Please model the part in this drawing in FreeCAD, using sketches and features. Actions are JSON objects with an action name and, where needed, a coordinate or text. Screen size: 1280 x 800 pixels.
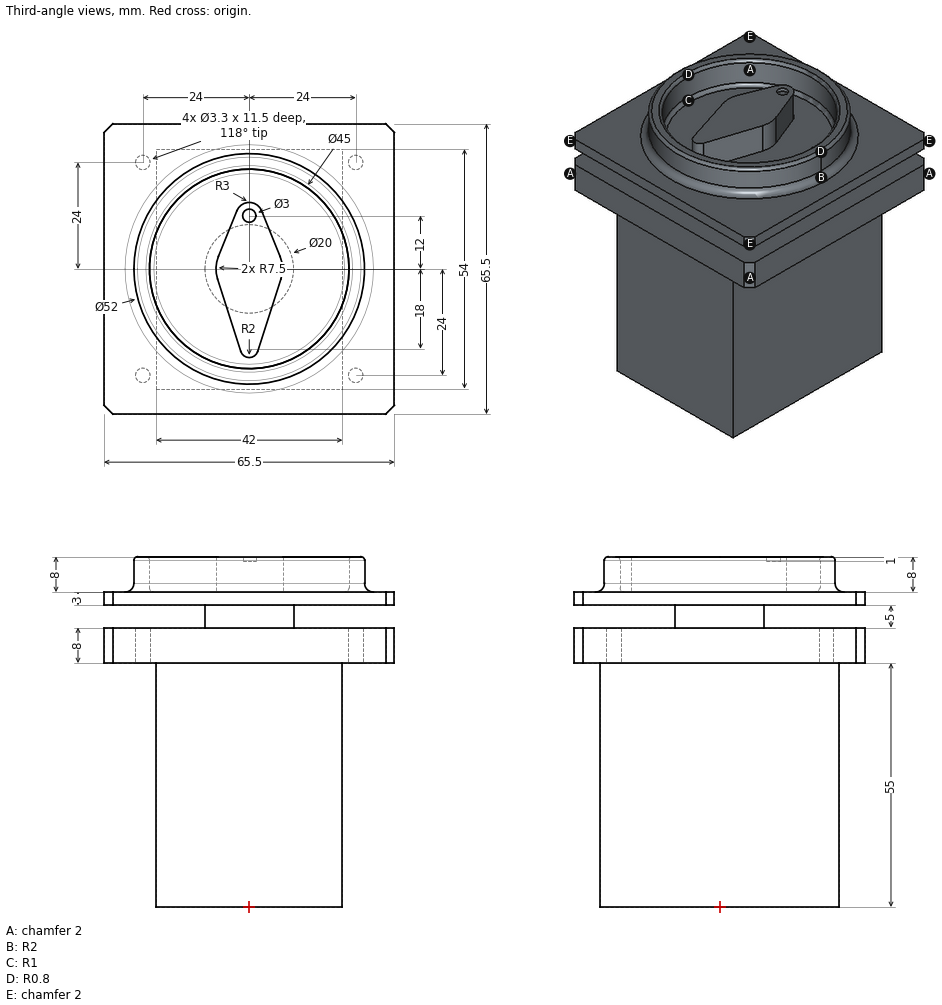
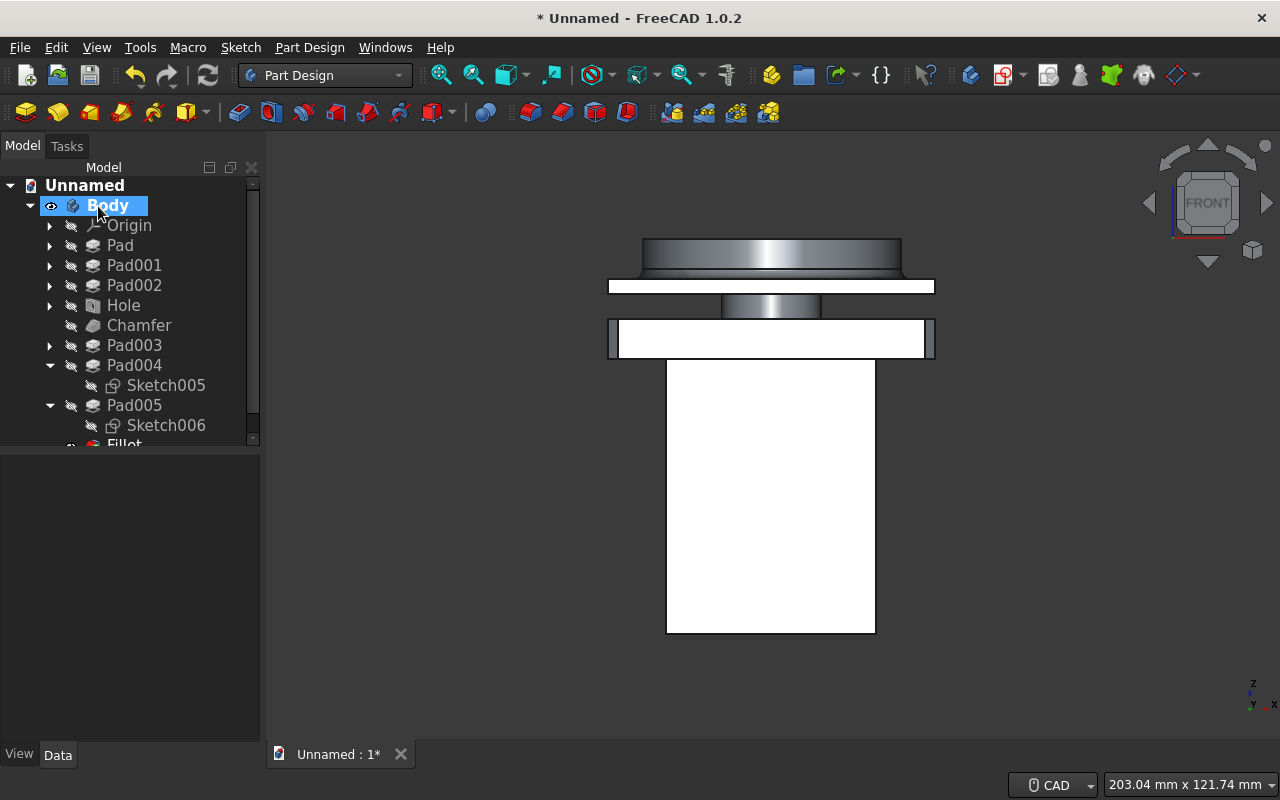
{"action": "key", "text": "3"}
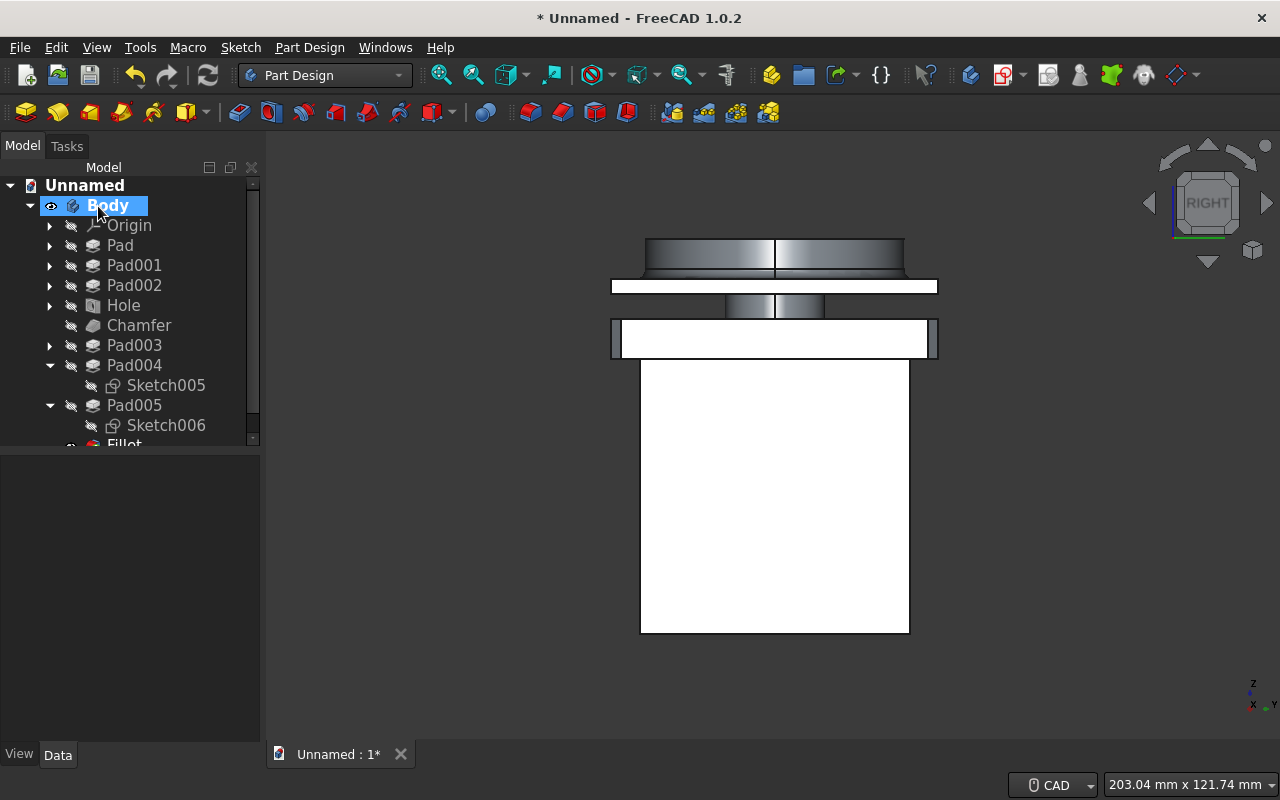
{"action": "key", "text": "5"}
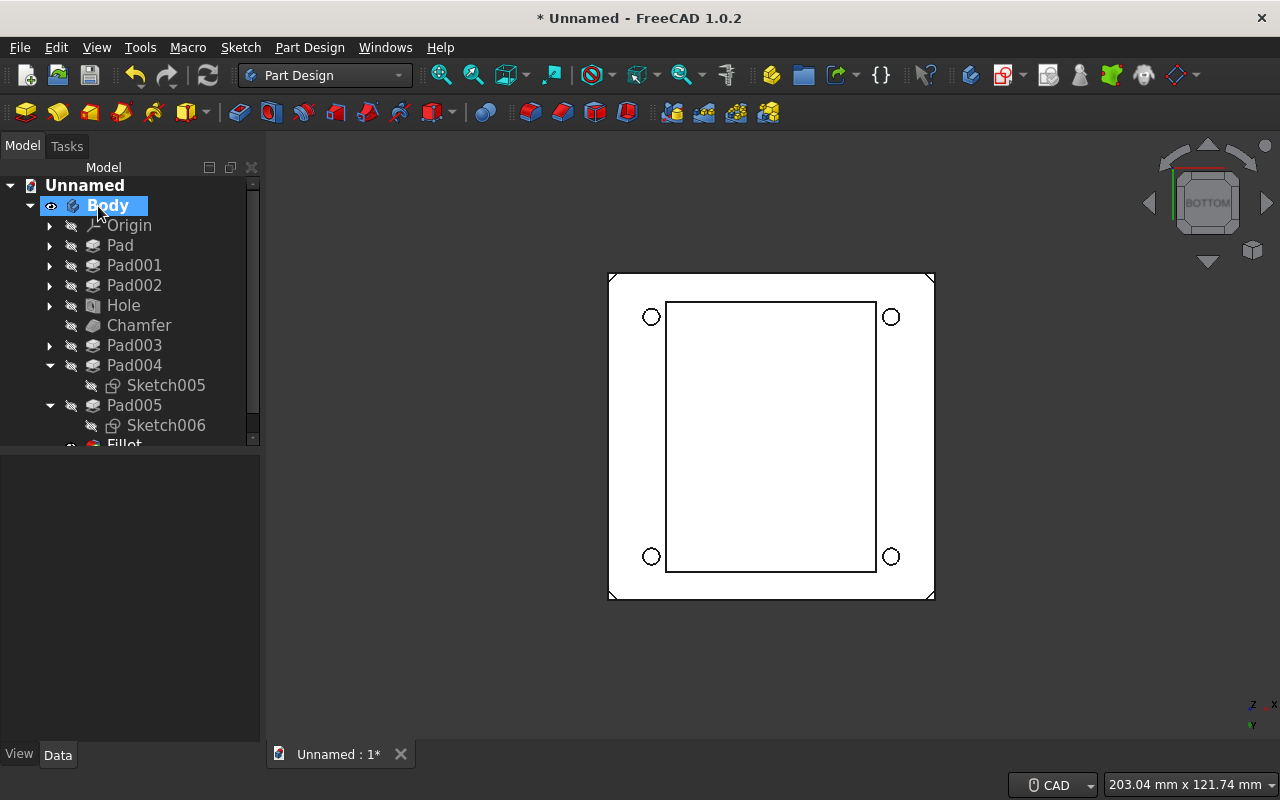
{"action": "key", "text": "4"}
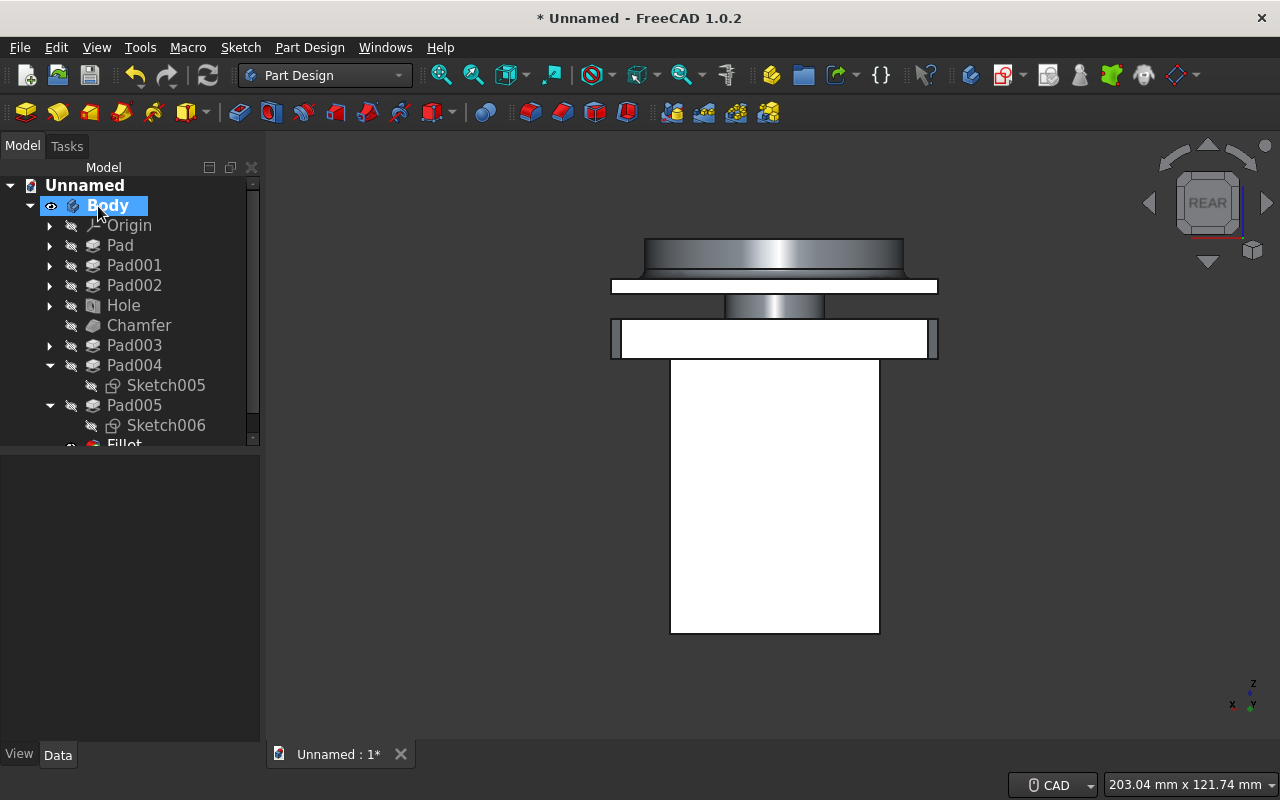
{"action": "key", "text": "6"}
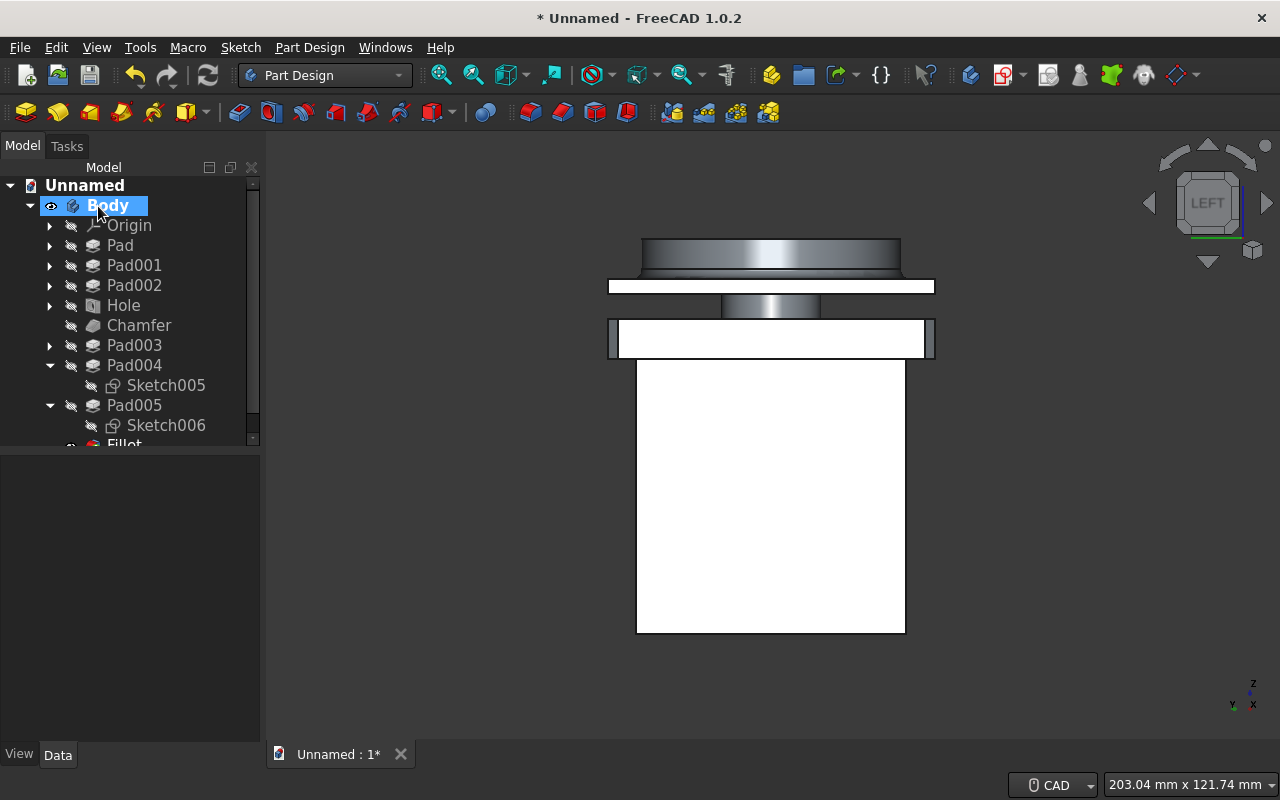
{"action": "key", "text": "v 3"}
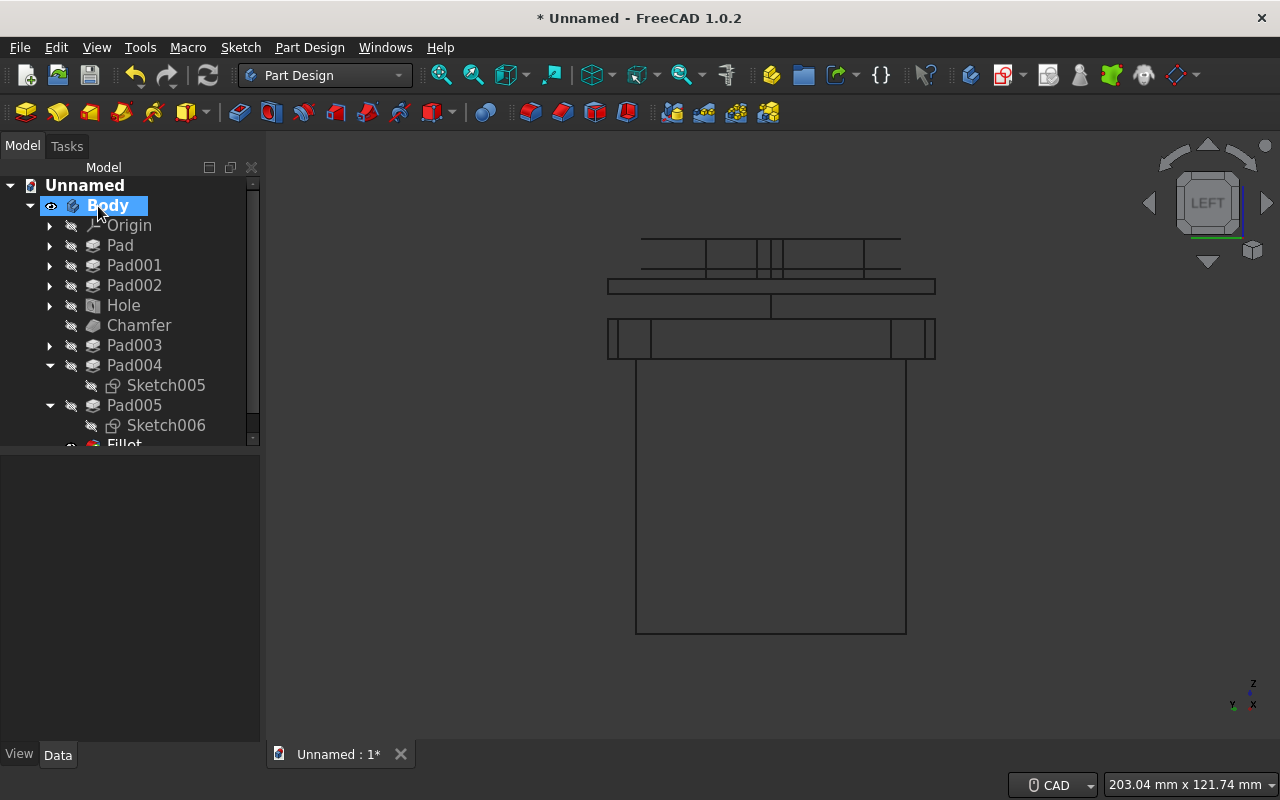
{"action": "key", "text": "0"}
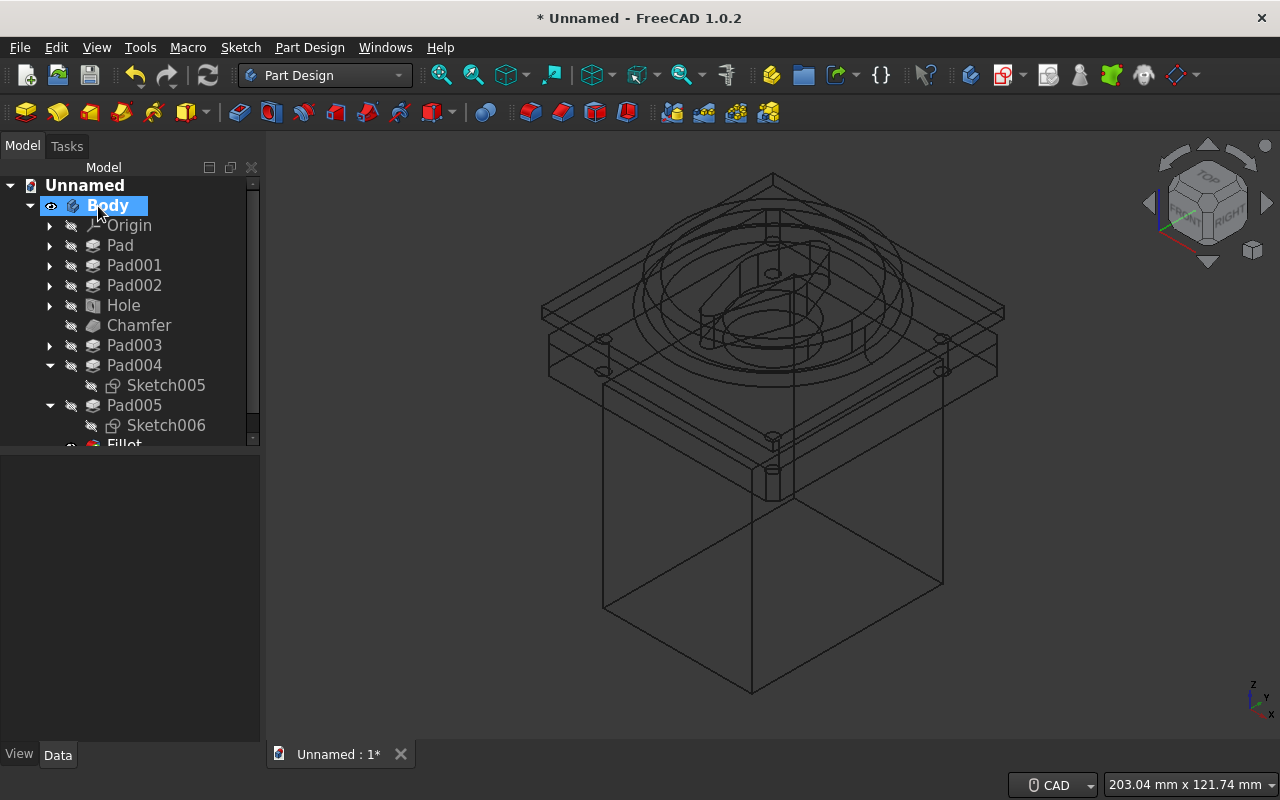
{"action": "left_click", "coordinate": [694, 260]}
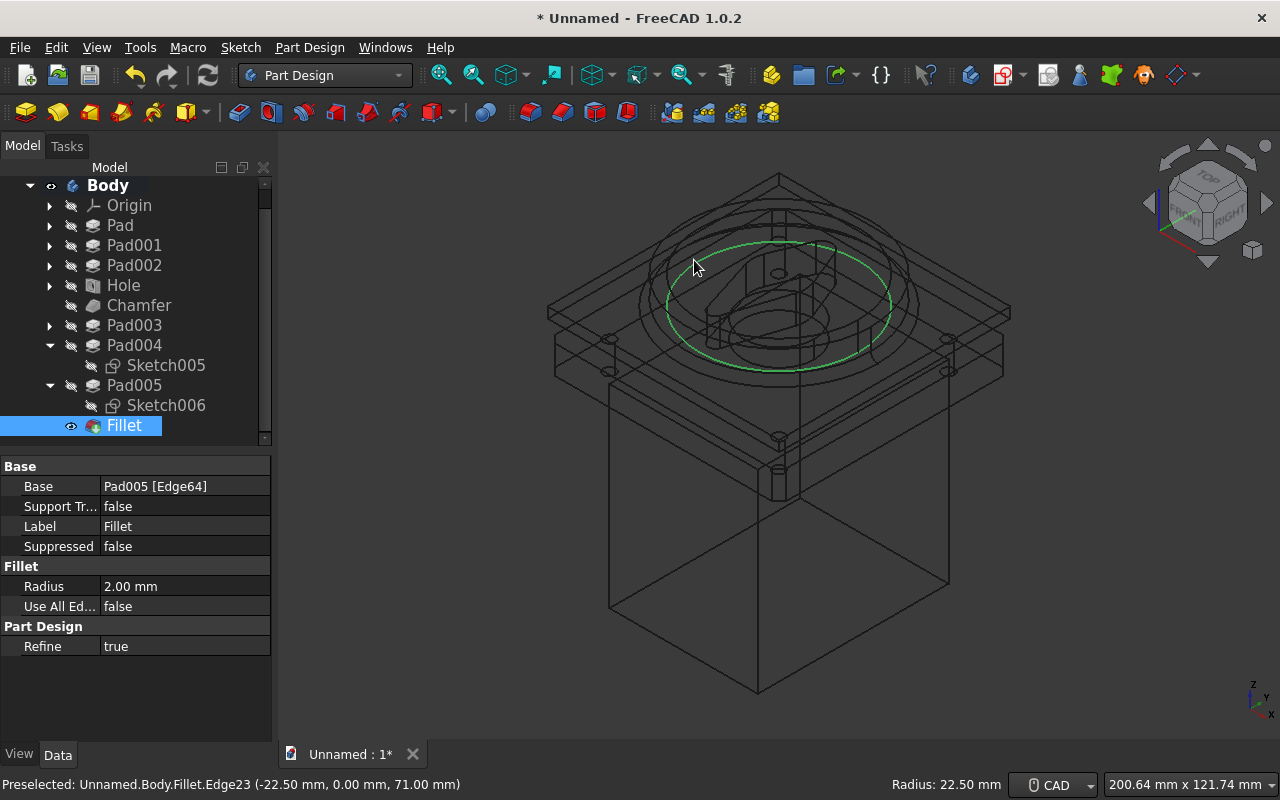
{"action": "key", "text": "v 1"}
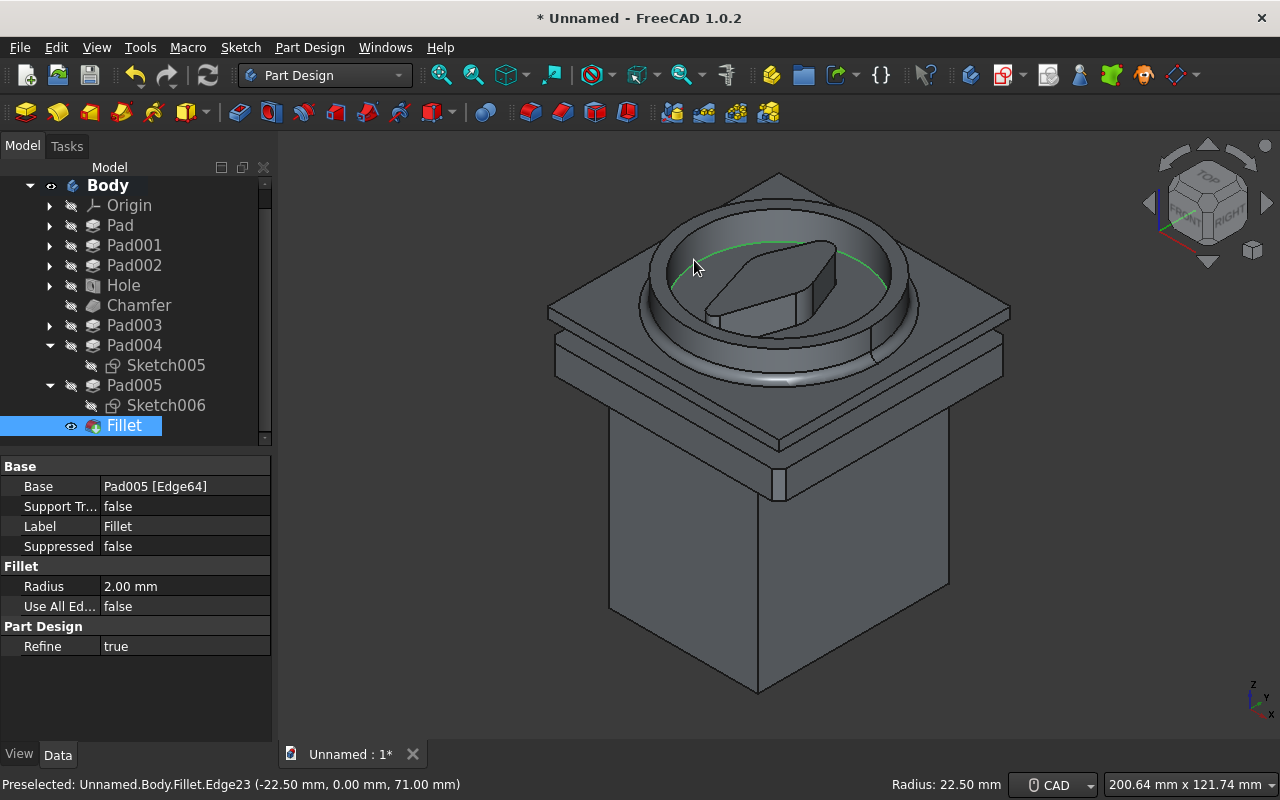
{"action": "left_click", "coordinate": [532, 112]}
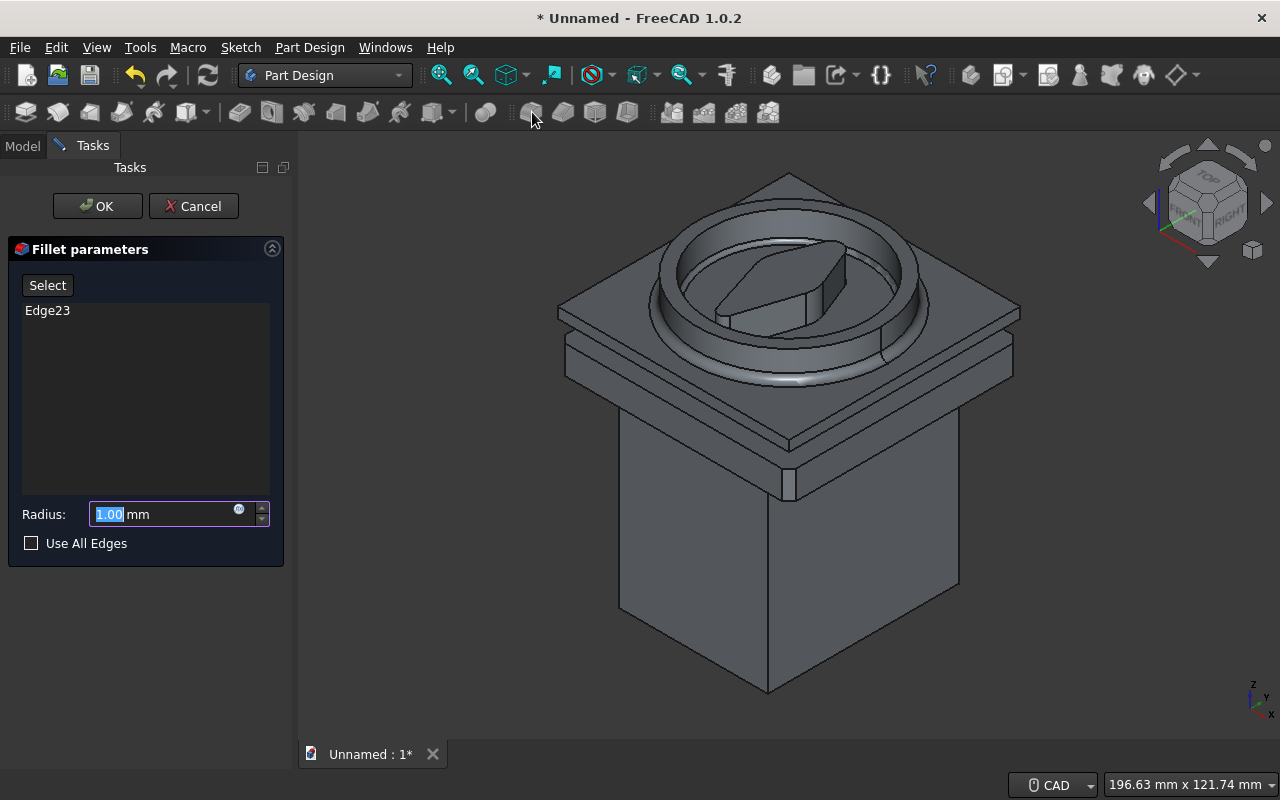
{"action": "type", "text": "1"}
{"action": "key", "text": "Tab"}